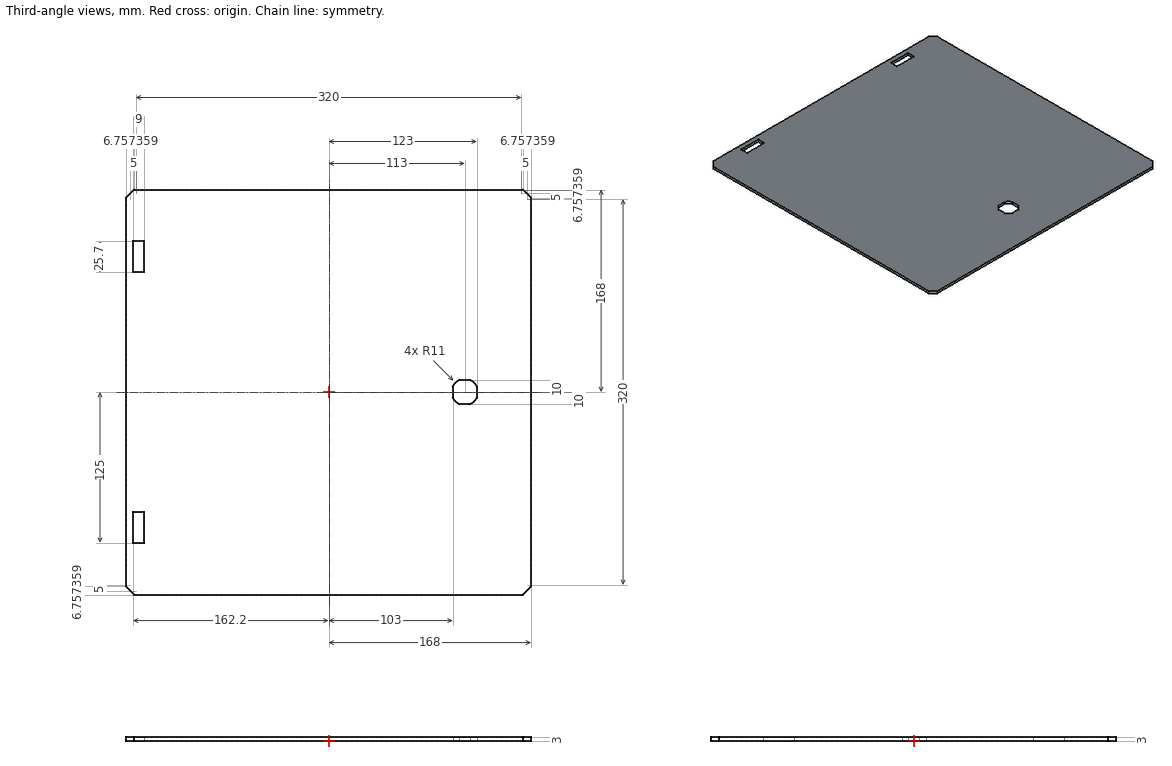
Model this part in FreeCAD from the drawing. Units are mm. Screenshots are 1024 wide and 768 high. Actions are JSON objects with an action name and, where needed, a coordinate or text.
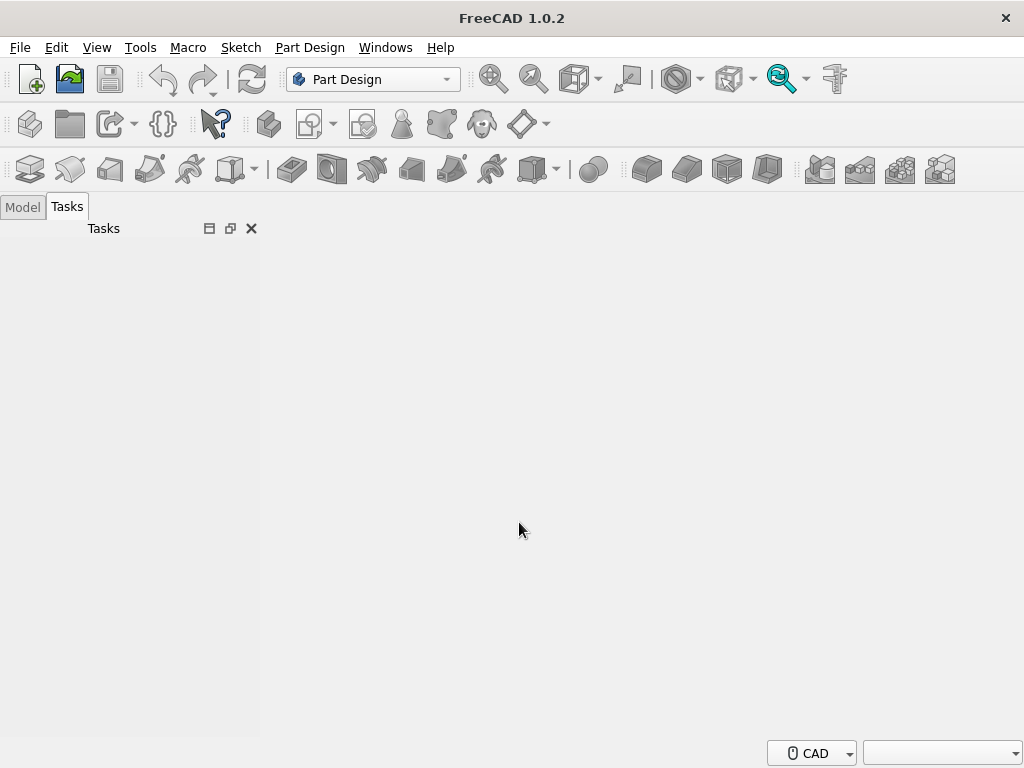
{"action": "left_click", "coordinate": [30, 80]}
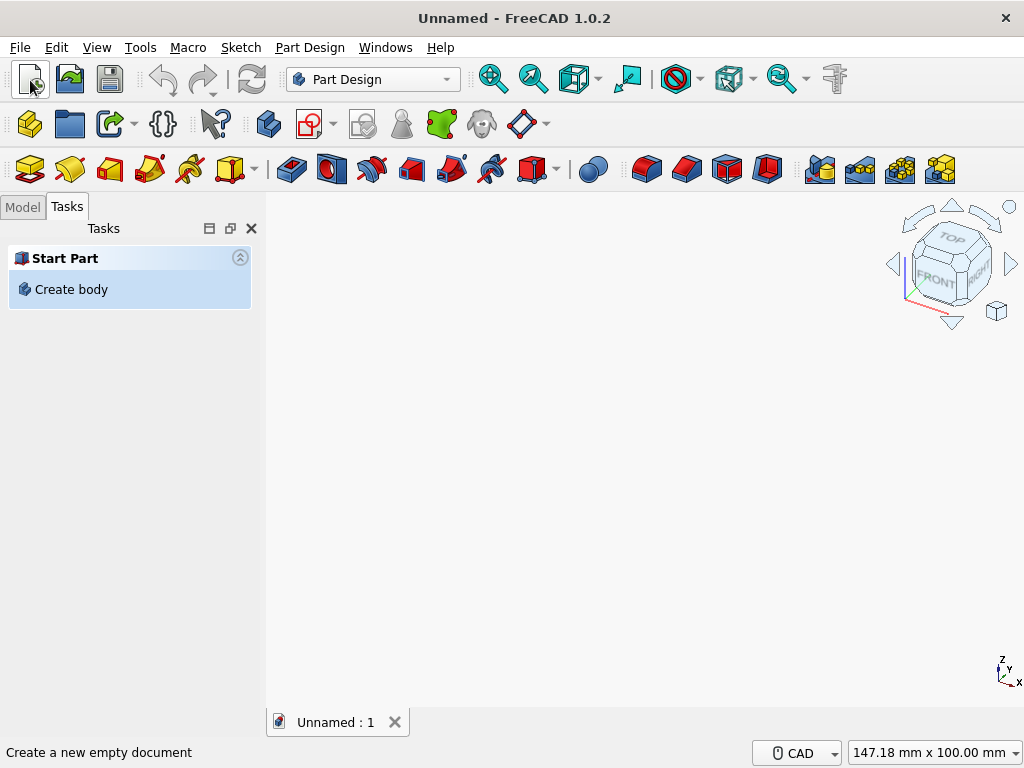
{"action": "left_click", "coordinate": [310, 124]}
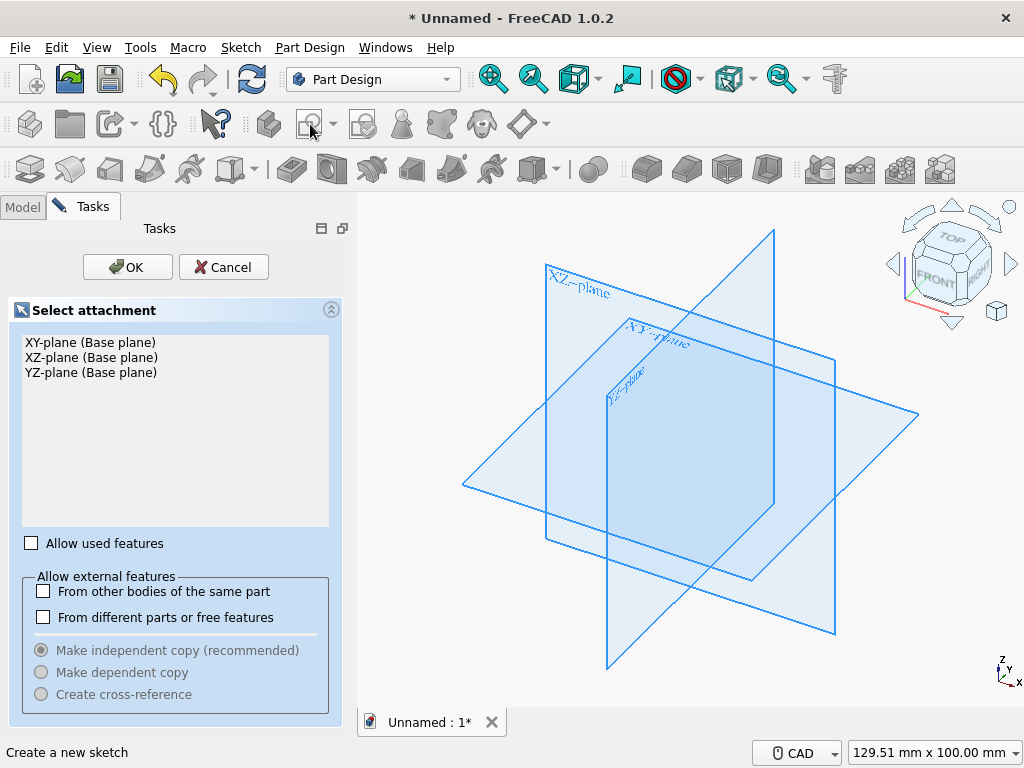
{"action": "left_click", "coordinate": [82, 342]}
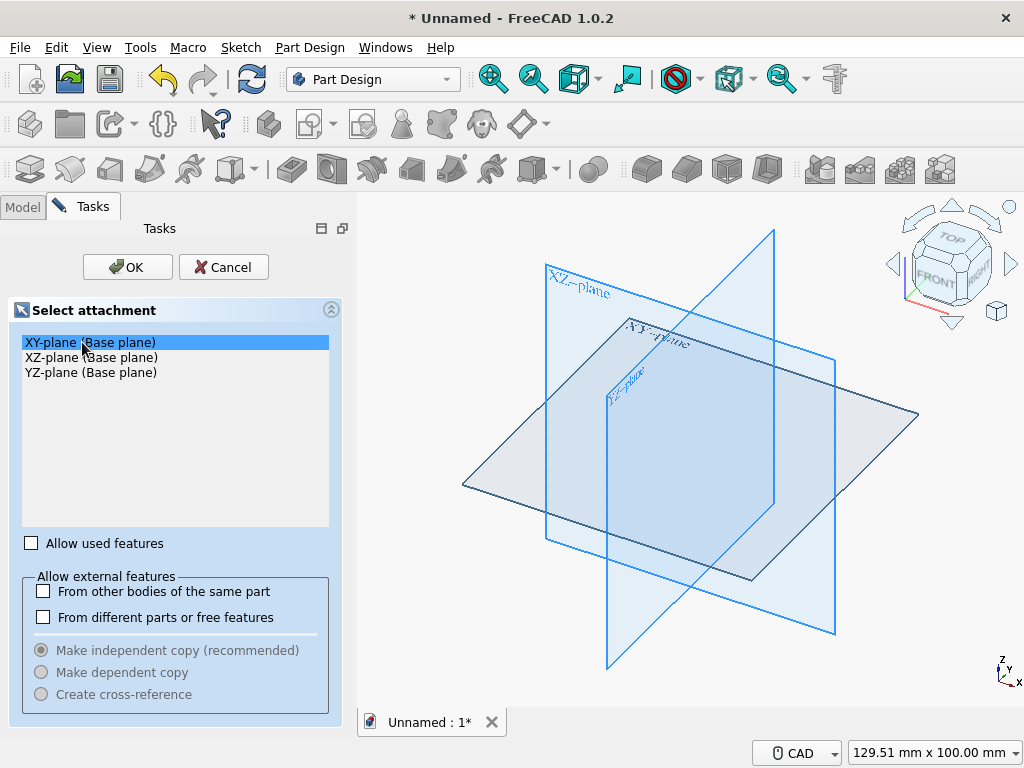
{"action": "left_click", "coordinate": [128, 267]}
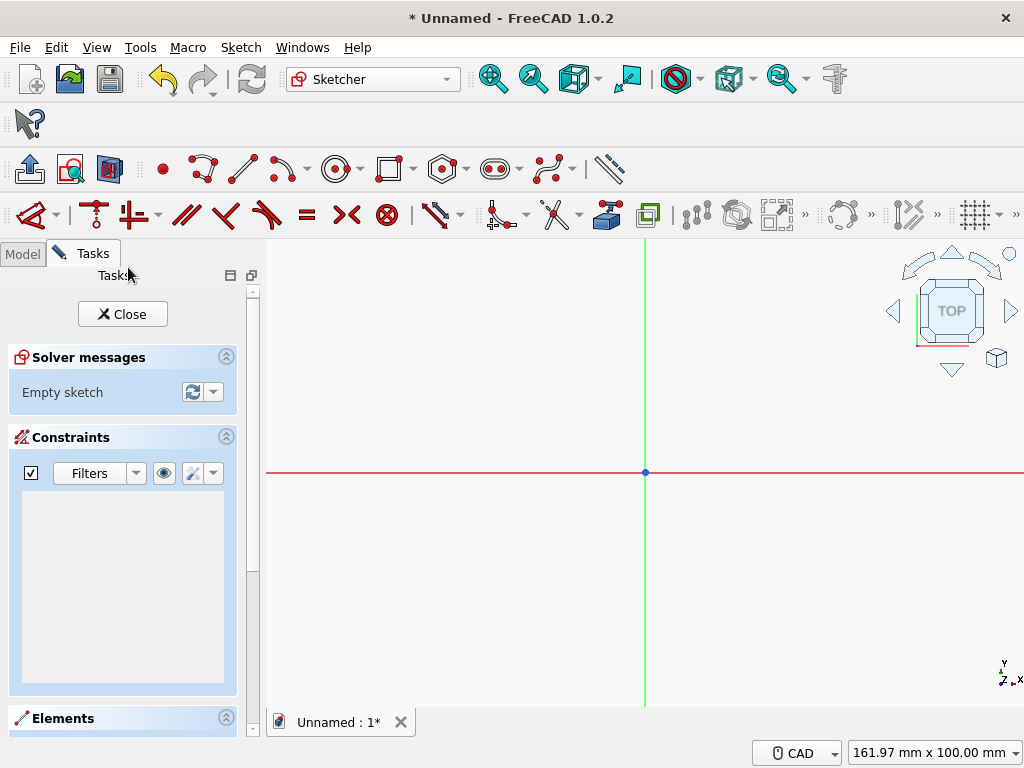
{"action": "scroll", "coordinate": [559, 473], "scroll_direction": "down", "scroll_amount": 8}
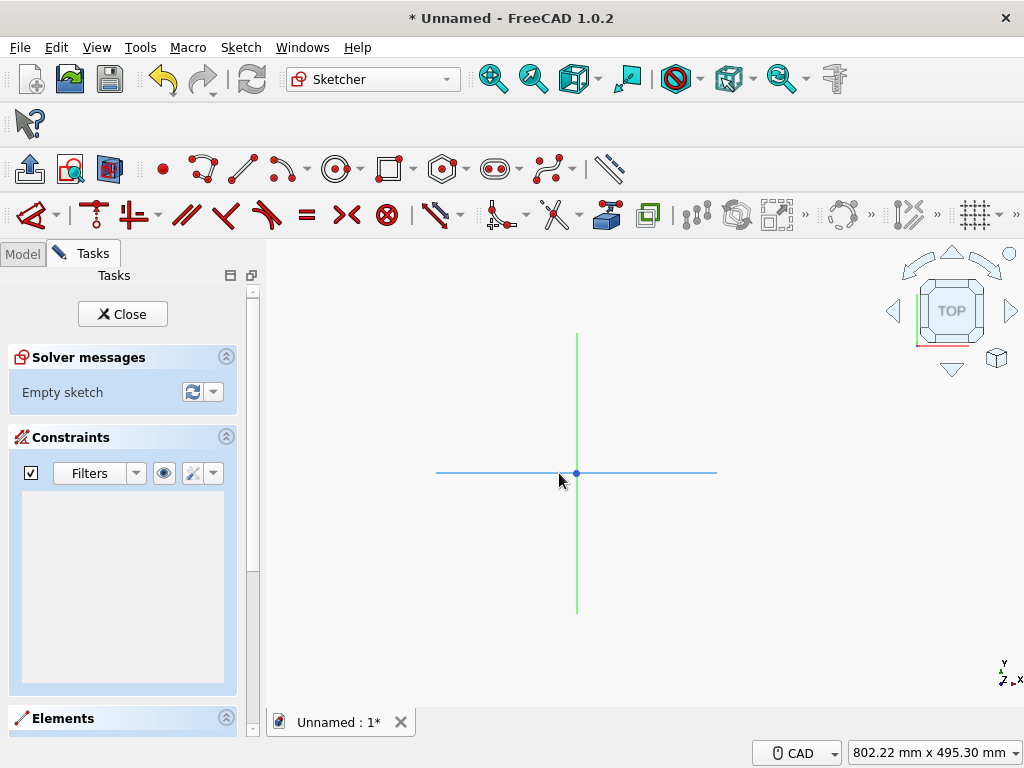
{"action": "left_click", "coordinate": [204, 170]}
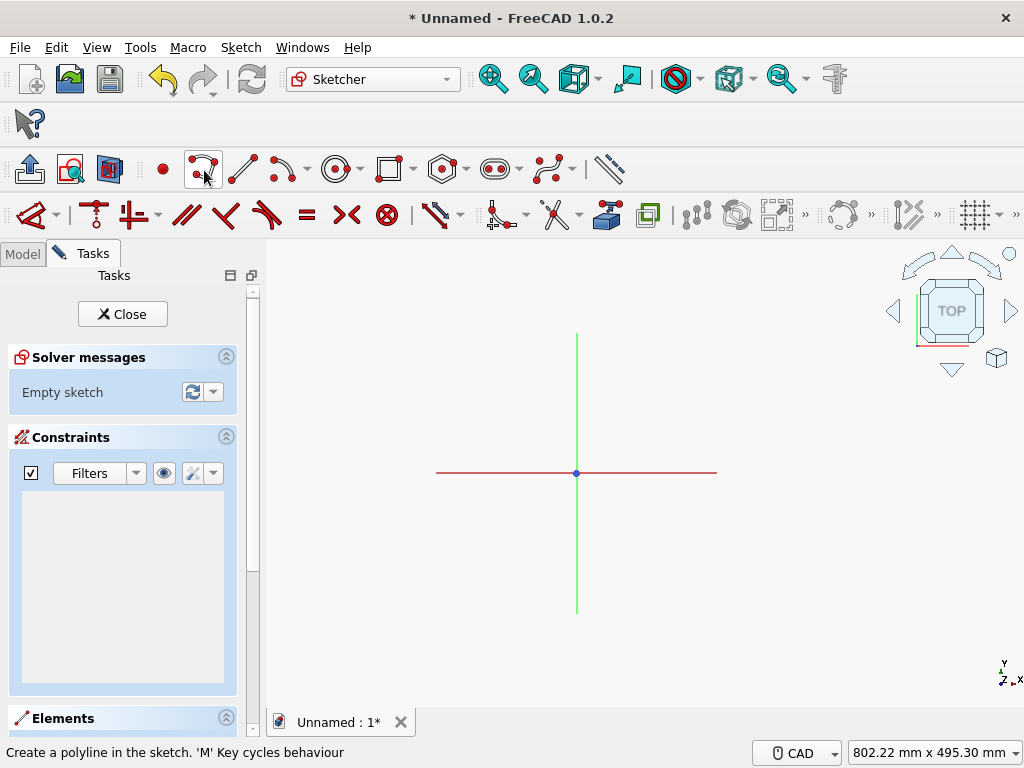
{"action": "left_click", "coordinate": [733, 625]}
{"action": "left_click", "coordinate": [733, 322]}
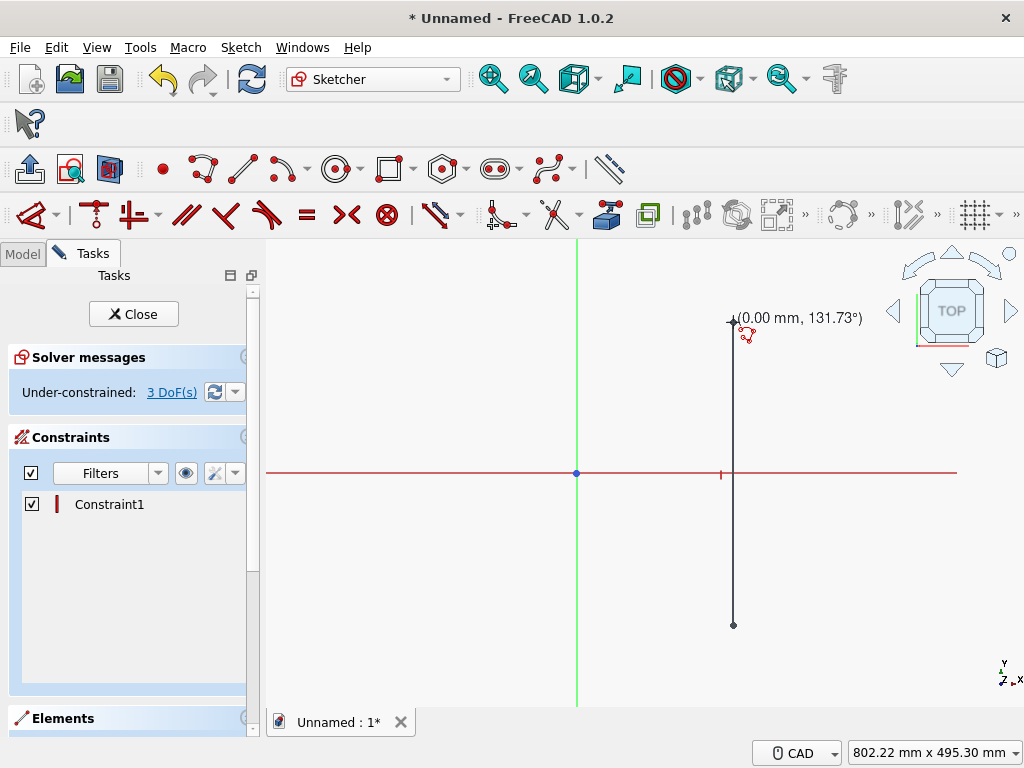
{"action": "scroll", "coordinate": [728, 317], "scroll_direction": "up", "scroll_amount": 5}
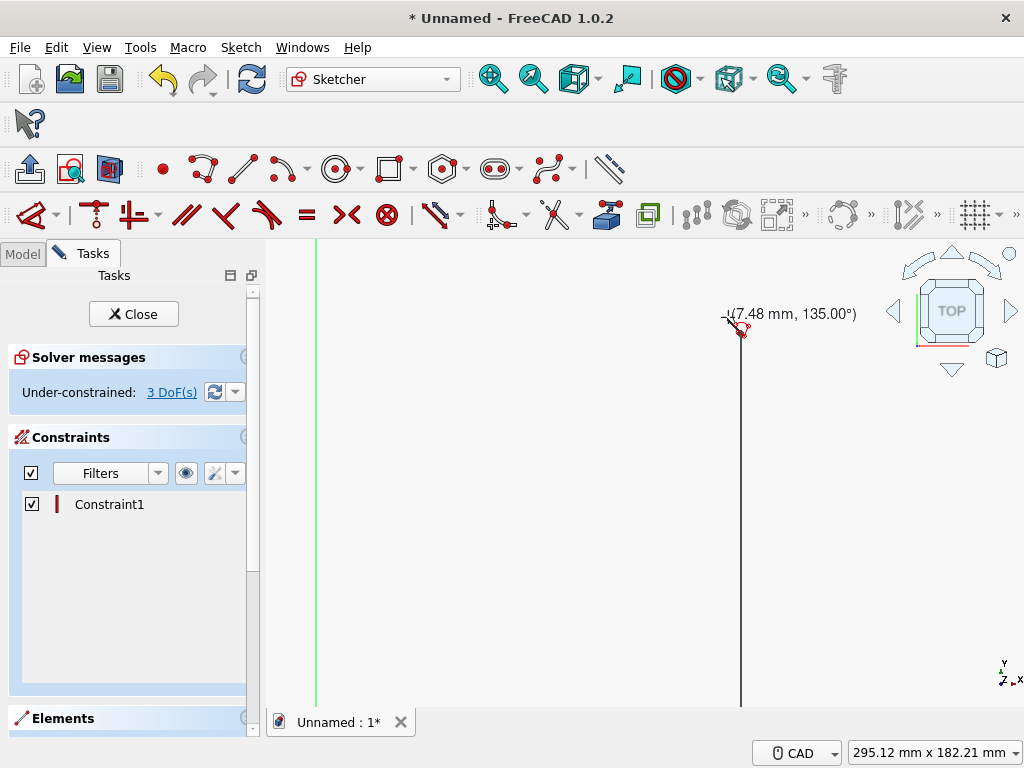
{"action": "left_click", "coordinate": [727, 318]}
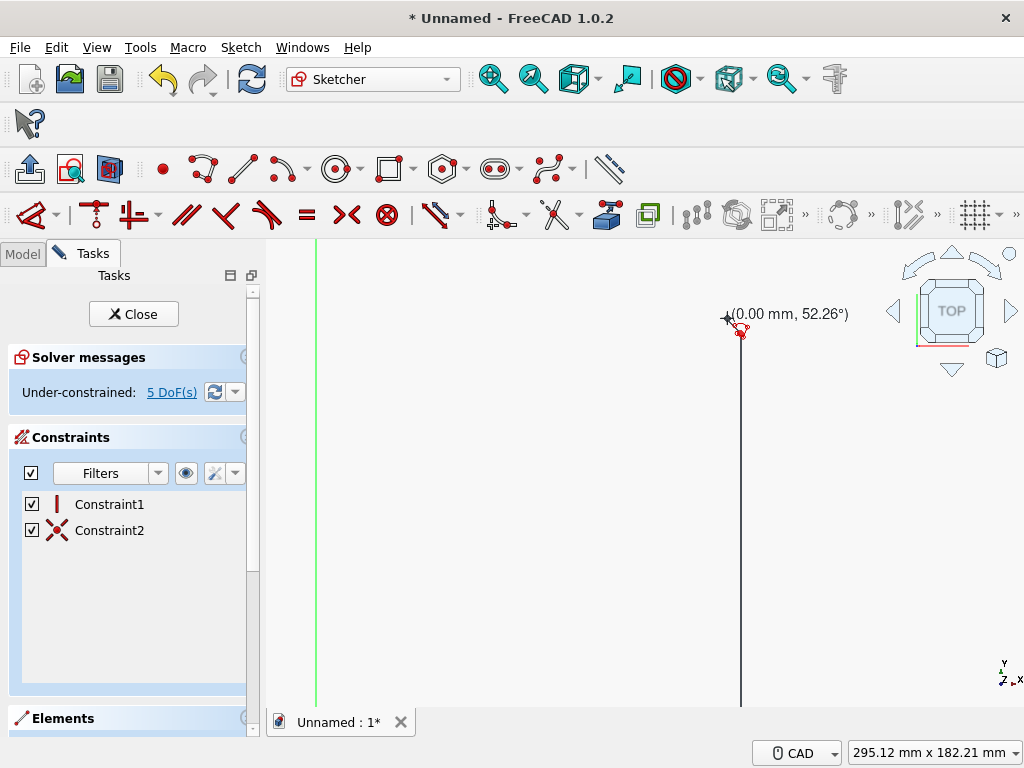
{"action": "scroll", "coordinate": [728, 317], "scroll_direction": "down", "scroll_amount": 5}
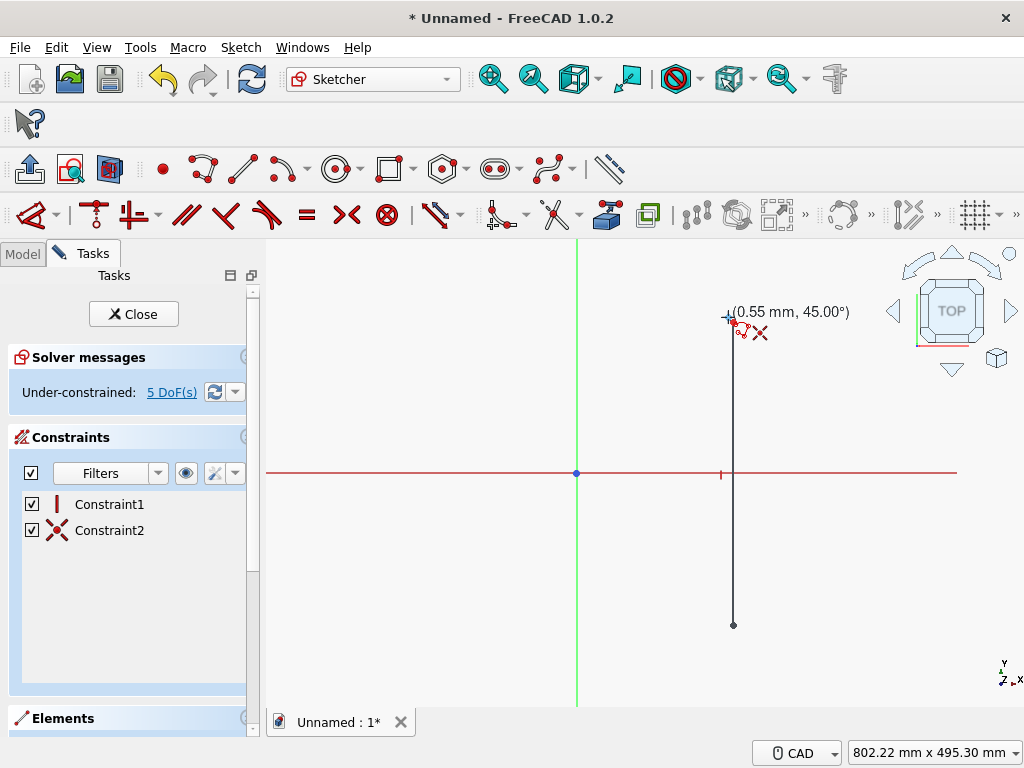
{"action": "left_click", "coordinate": [425, 317]}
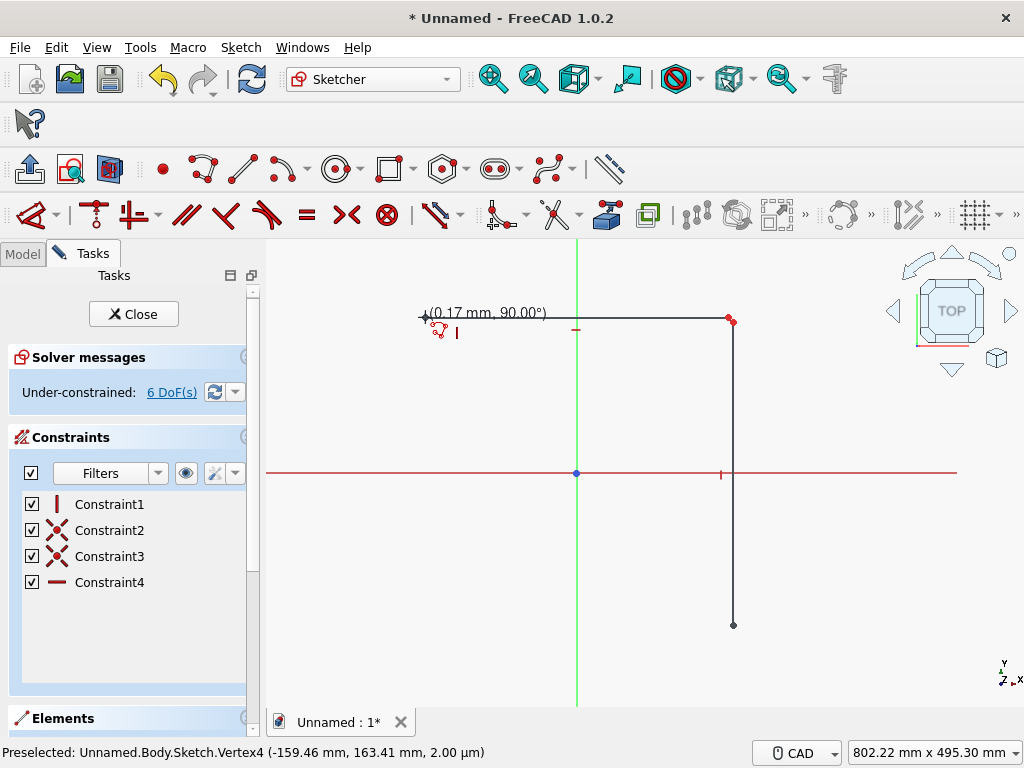
{"action": "scroll", "coordinate": [421, 322], "scroll_direction": "up", "scroll_amount": 5}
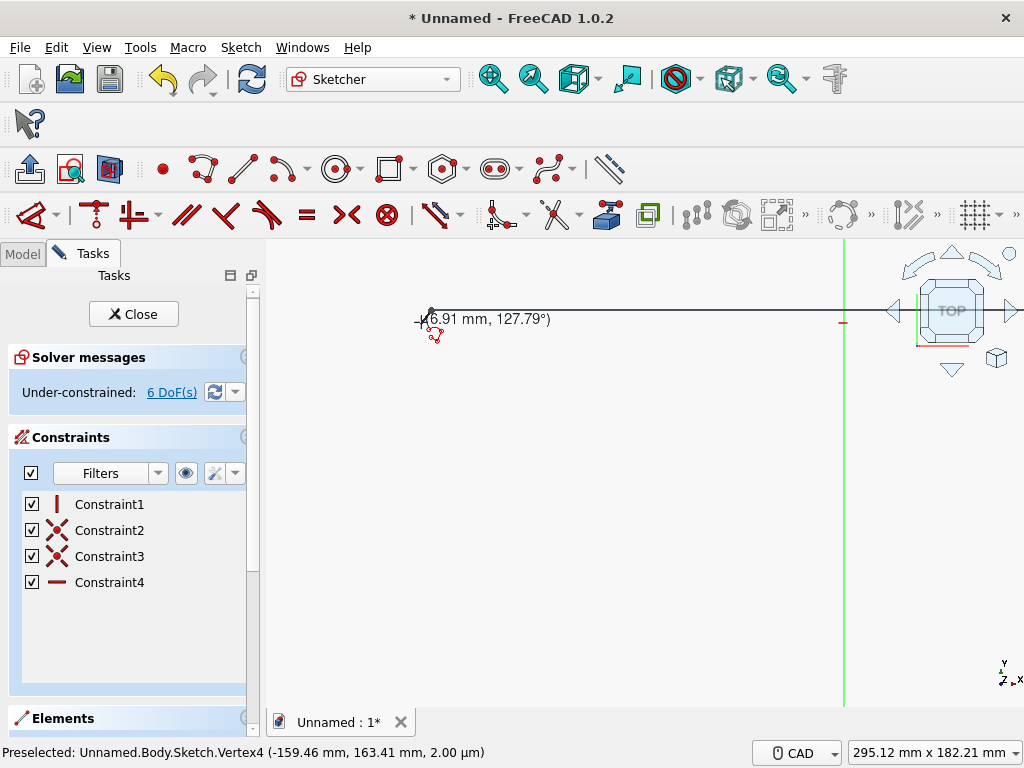
{"action": "left_click", "coordinate": [420, 322]}